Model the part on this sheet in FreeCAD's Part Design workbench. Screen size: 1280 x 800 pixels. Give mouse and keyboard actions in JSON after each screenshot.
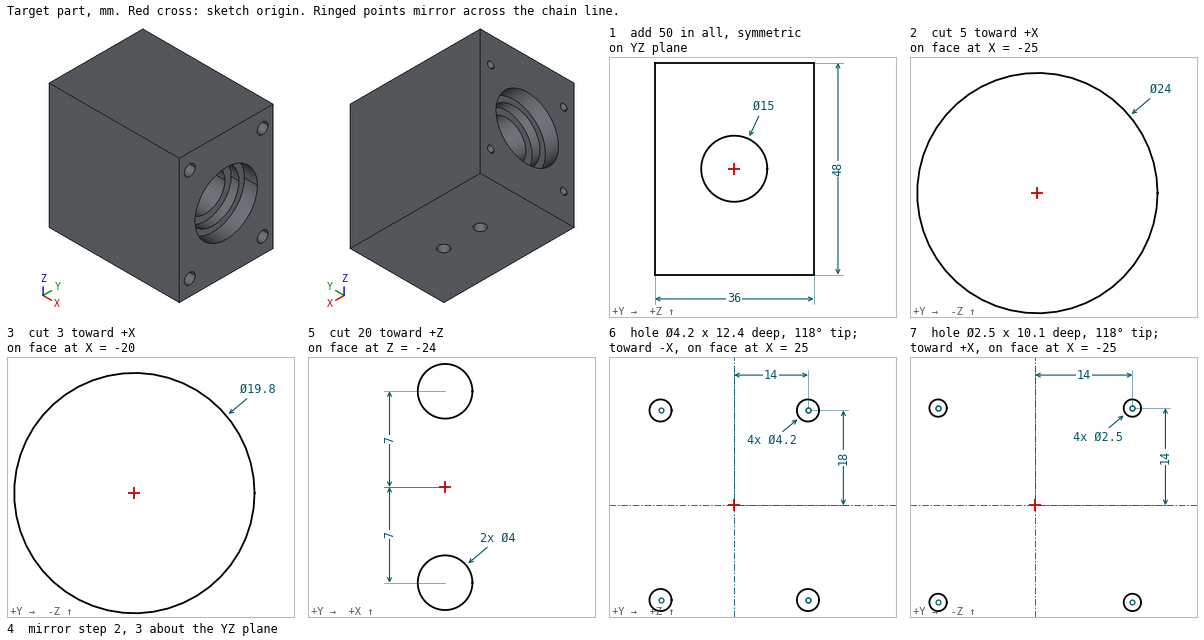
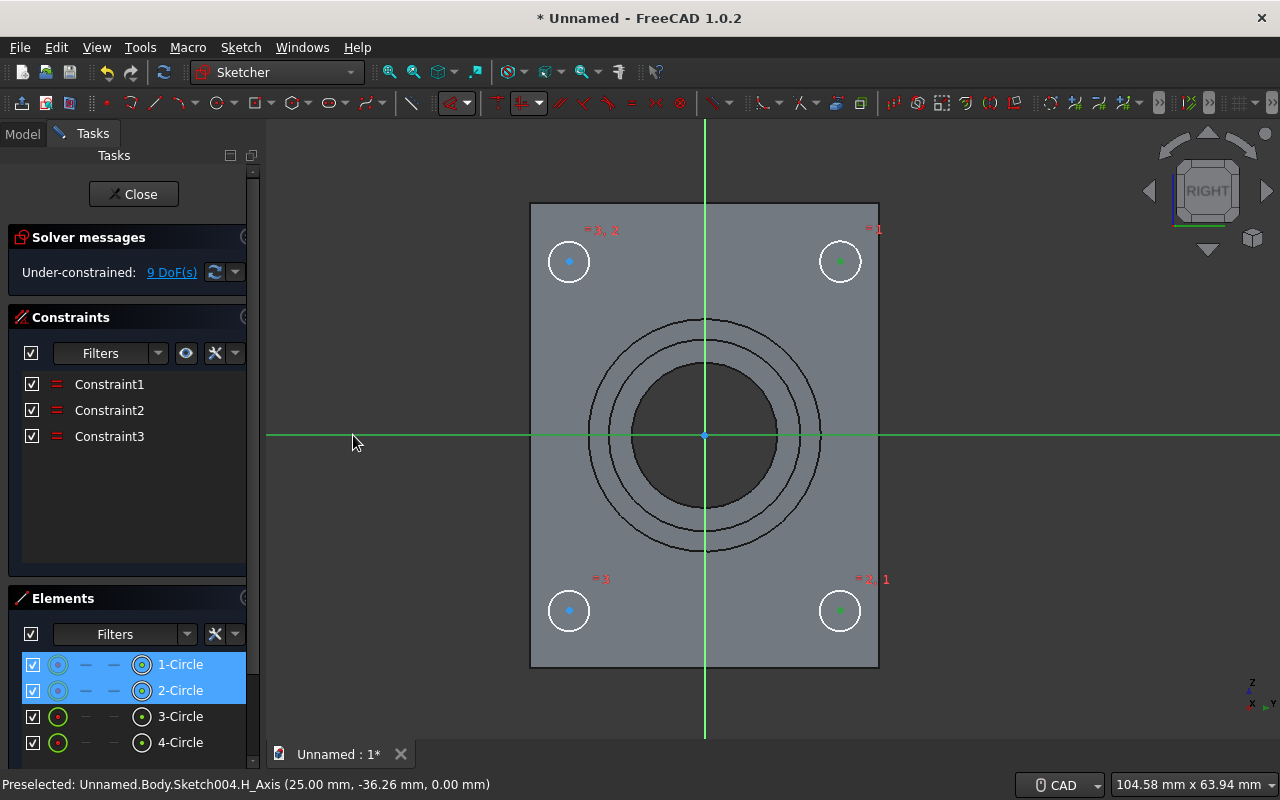
{"action": "left_click", "coordinate": [656, 104]}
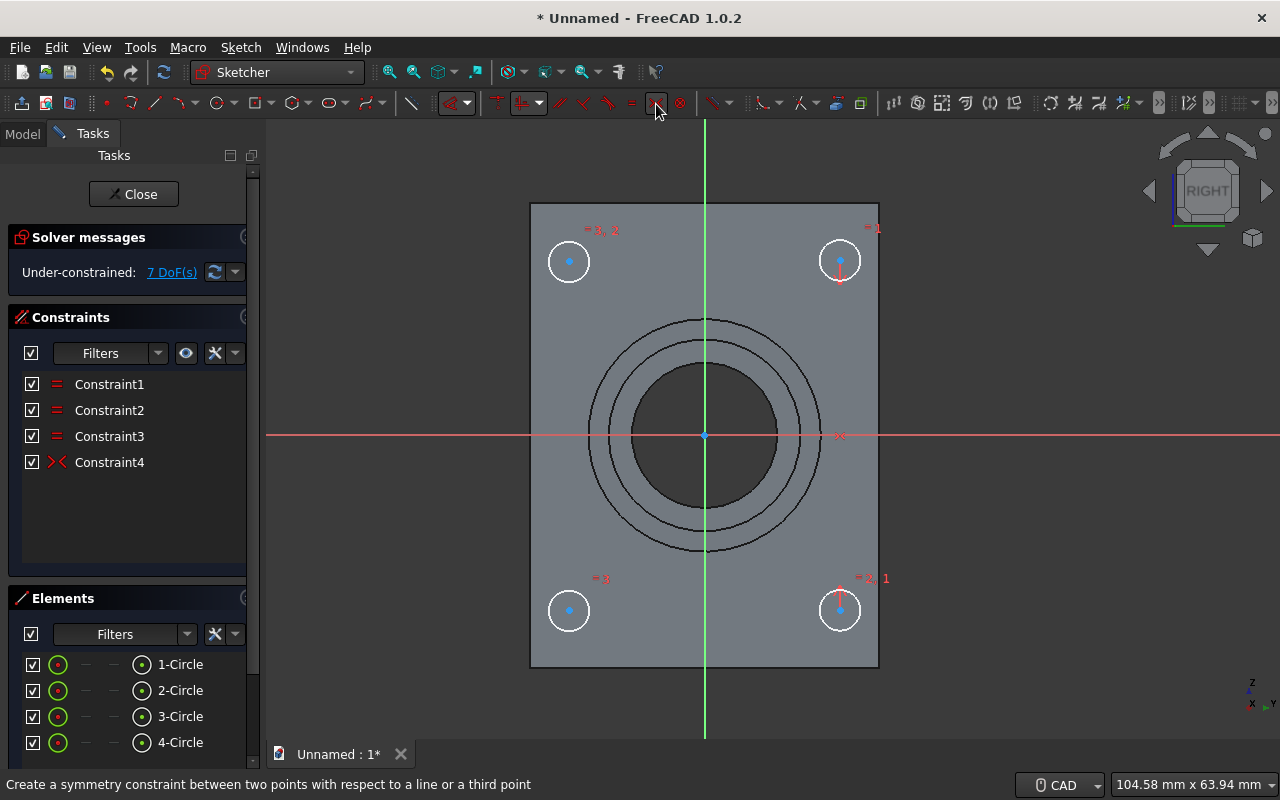
{"action": "left_click", "coordinate": [840, 260]}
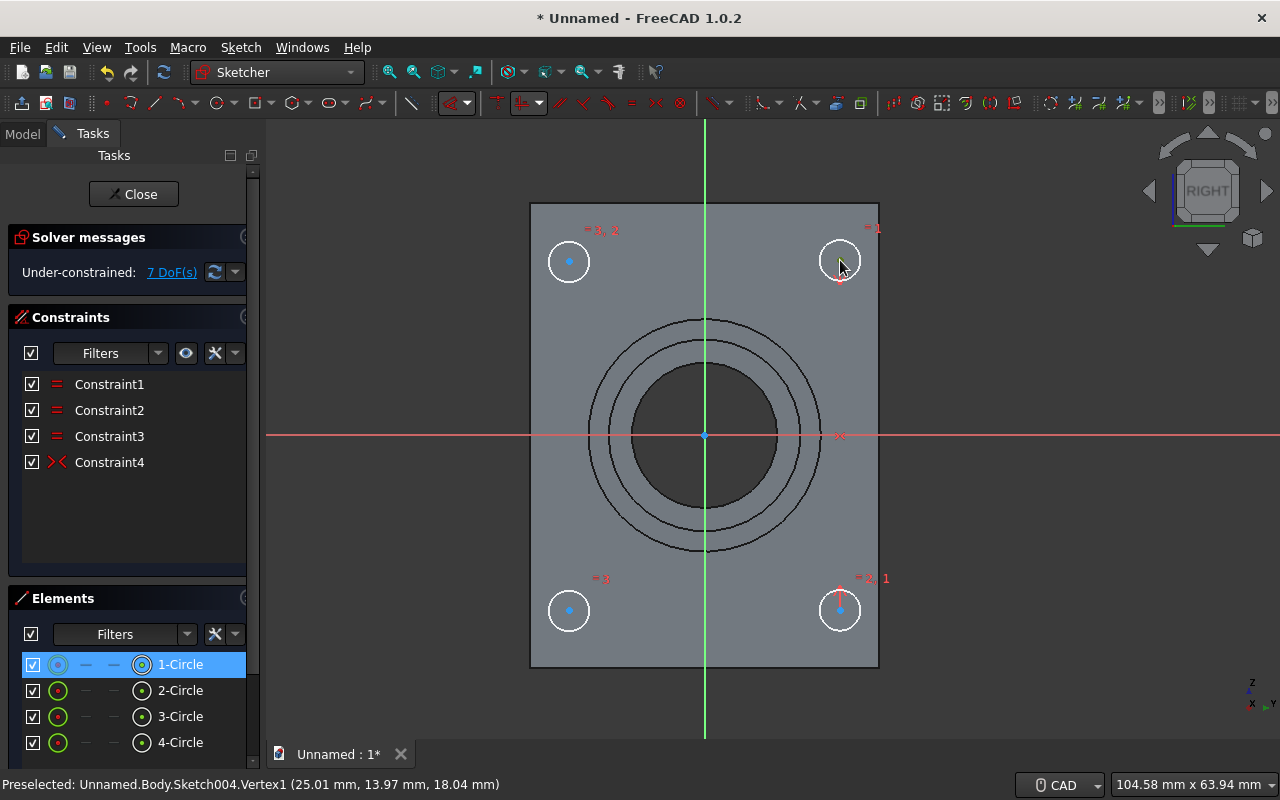
{"action": "left_click", "coordinate": [569, 262]}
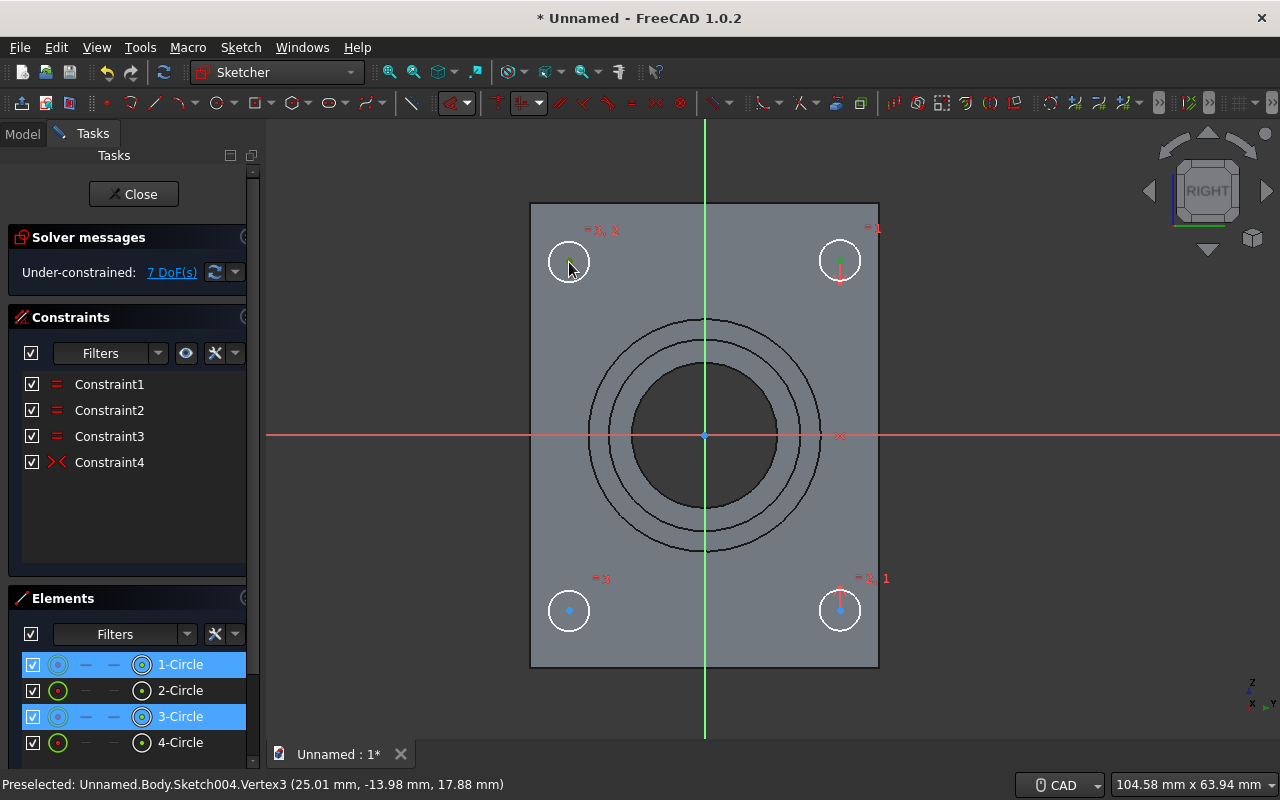
{"action": "left_click", "coordinate": [705, 671]}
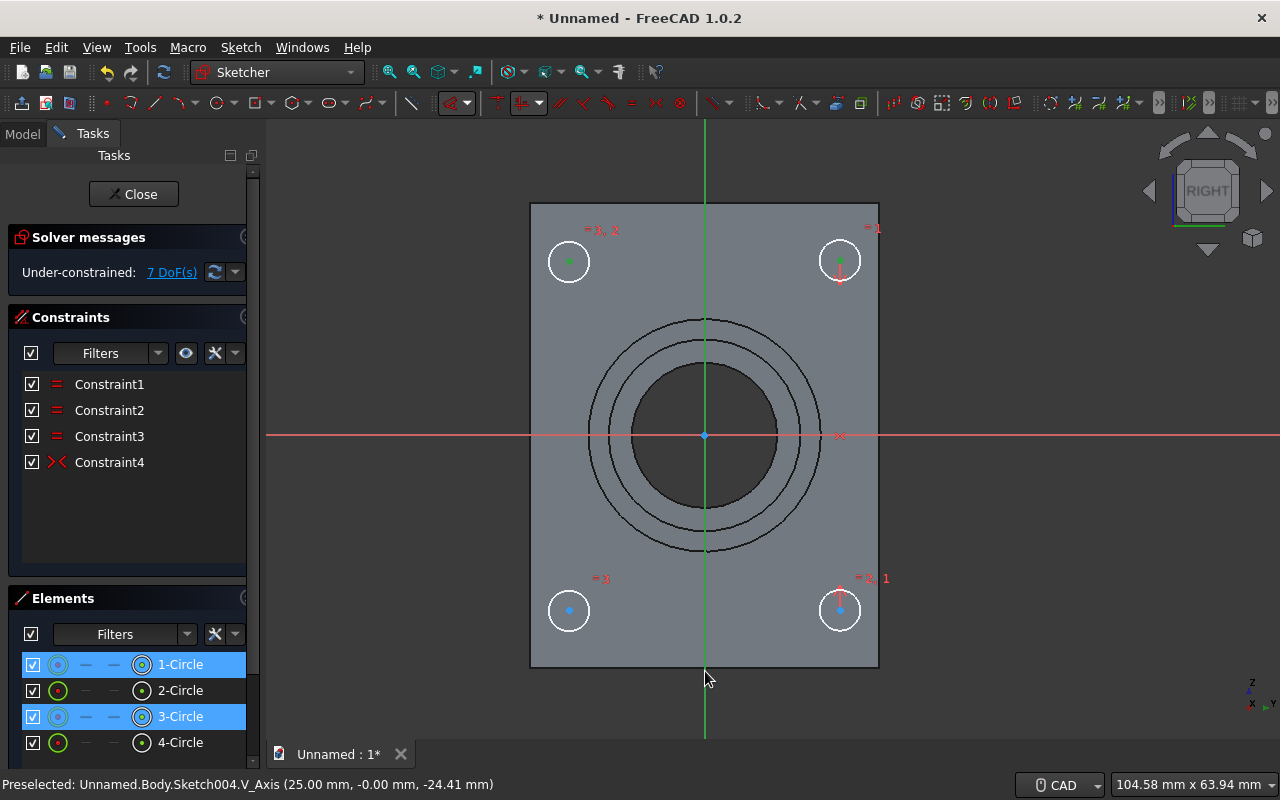
{"action": "left_click", "coordinate": [656, 104]}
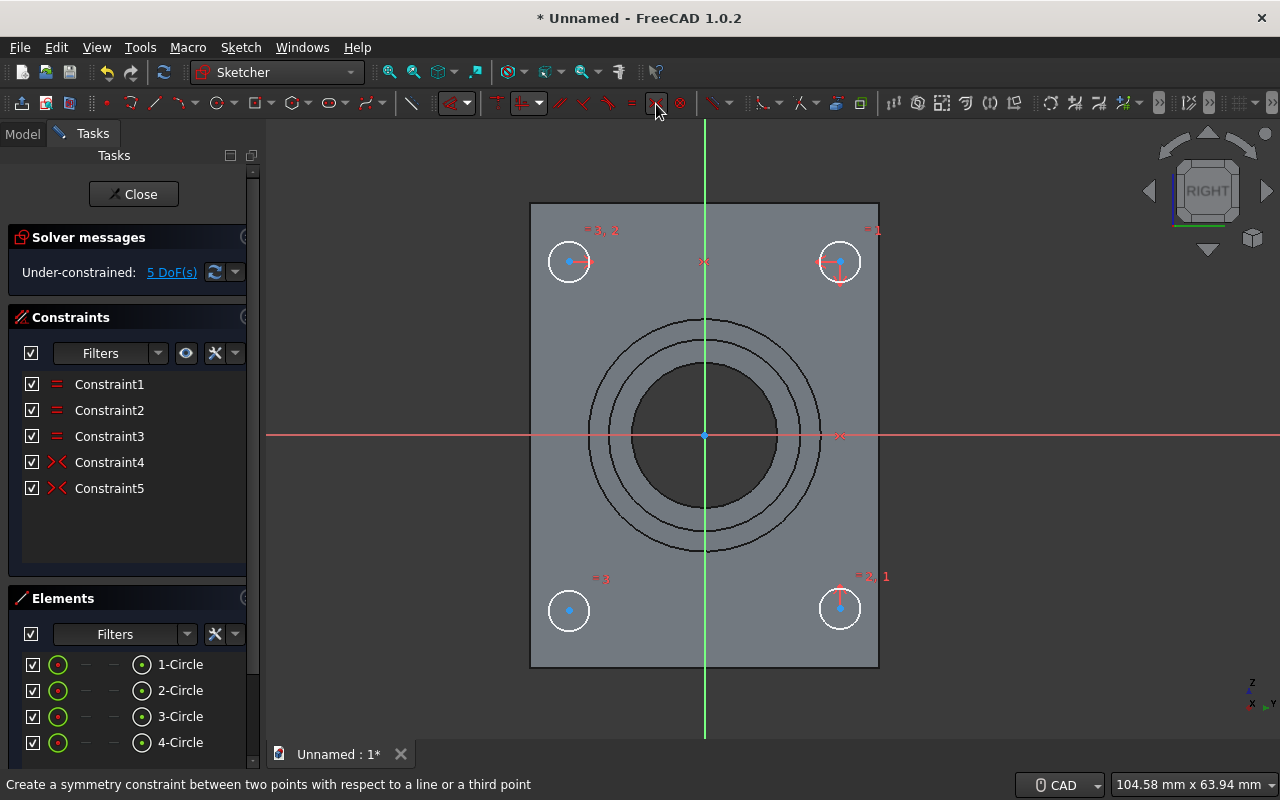
{"action": "left_click", "coordinate": [840, 609]}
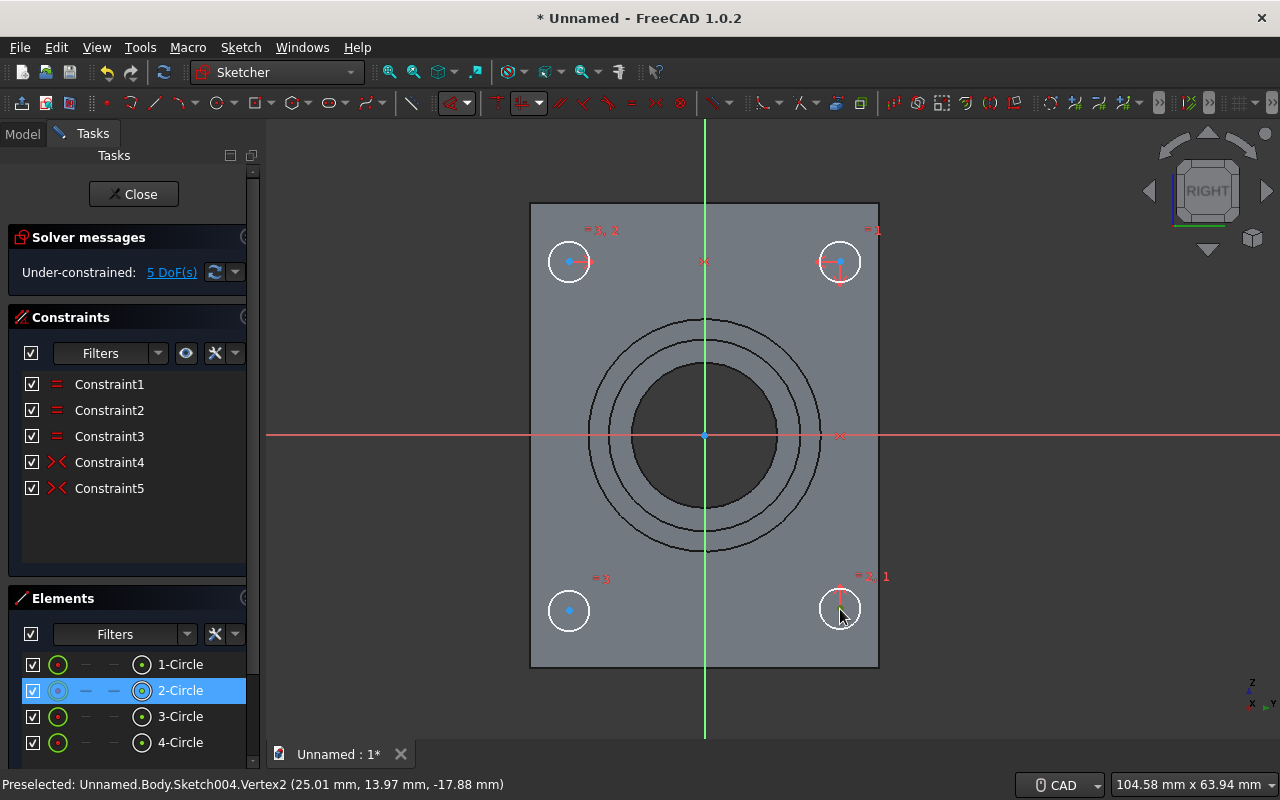
{"action": "left_click", "coordinate": [569, 611]}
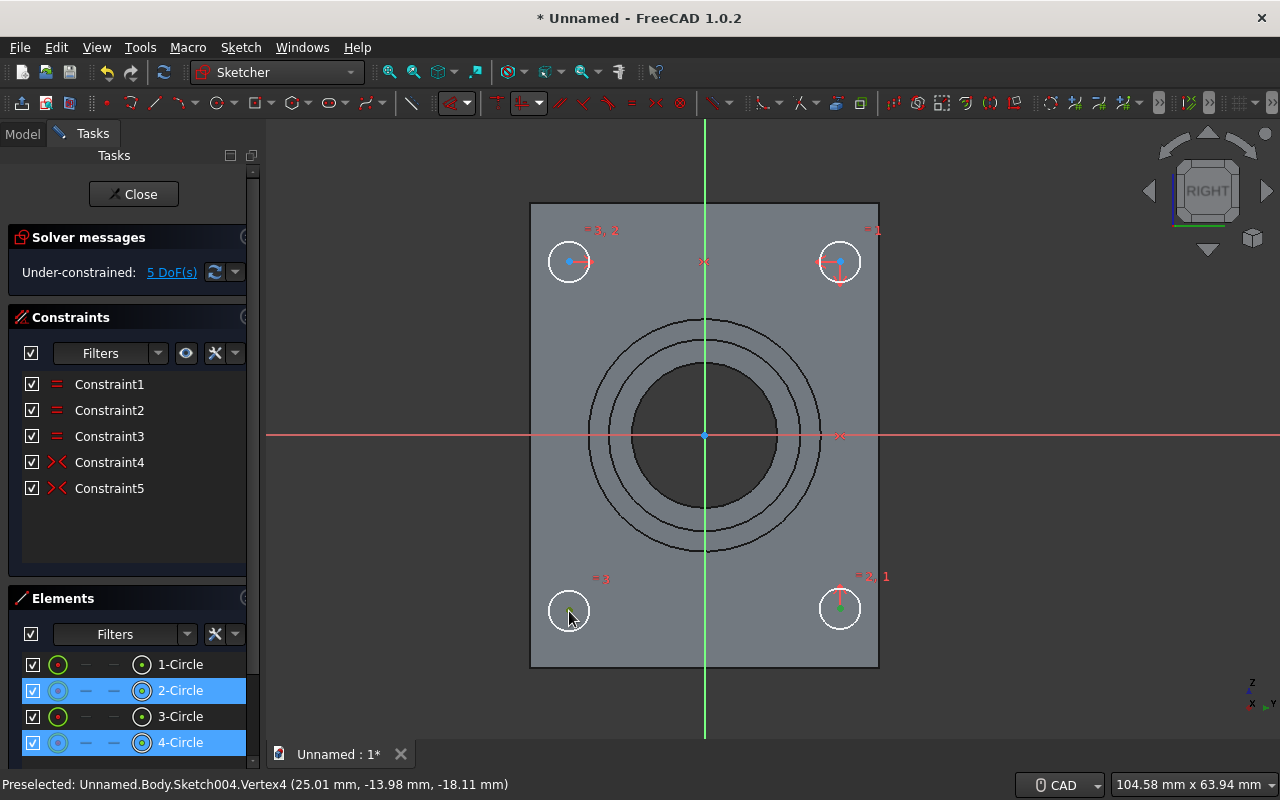
{"action": "left_click", "coordinate": [705, 671]}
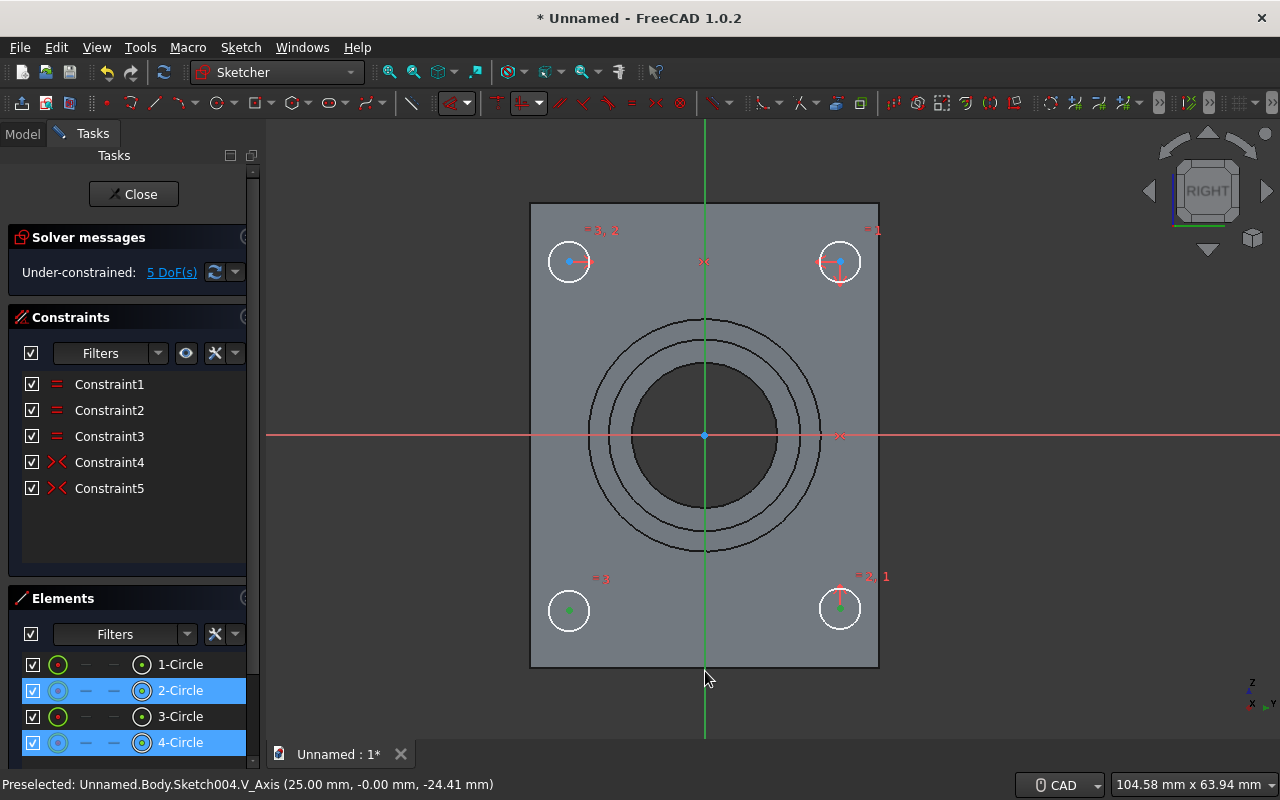
{"action": "left_click", "coordinate": [656, 104]}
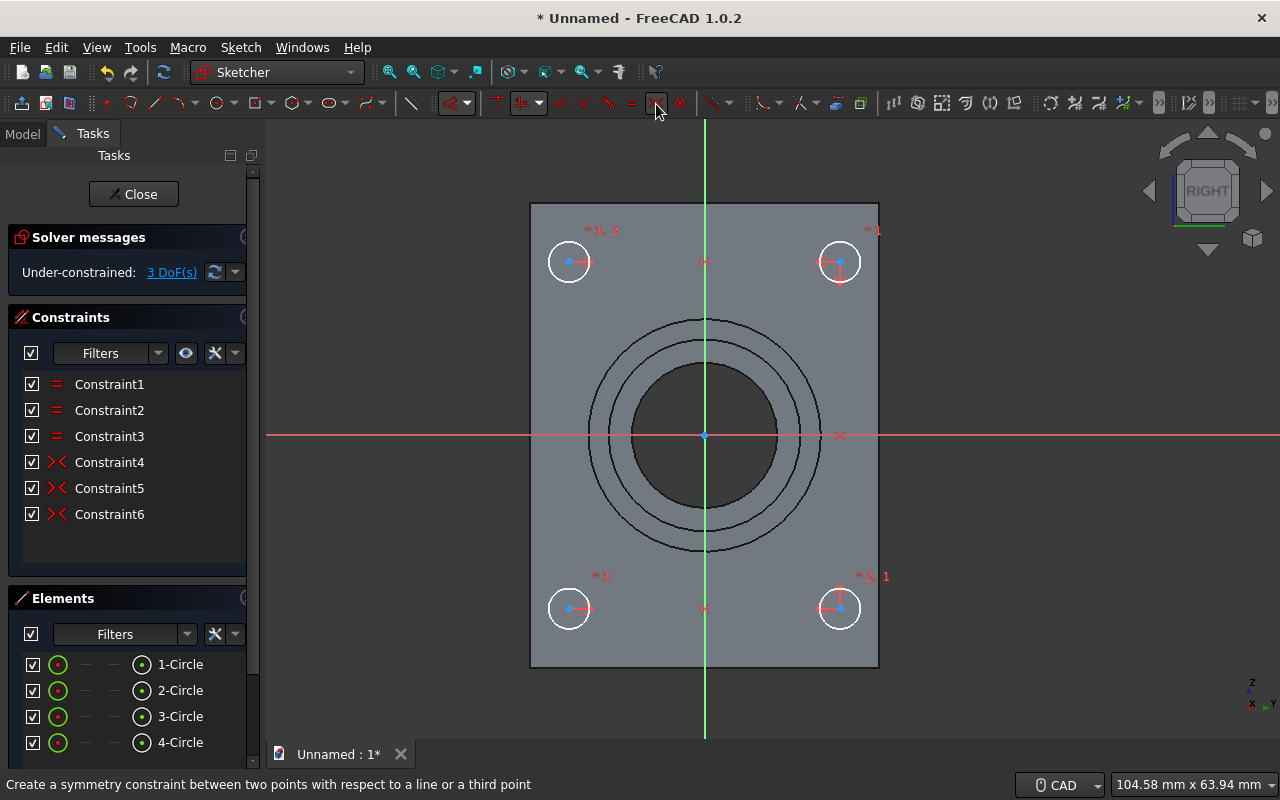
{"action": "left_click", "coordinate": [854, 248]}